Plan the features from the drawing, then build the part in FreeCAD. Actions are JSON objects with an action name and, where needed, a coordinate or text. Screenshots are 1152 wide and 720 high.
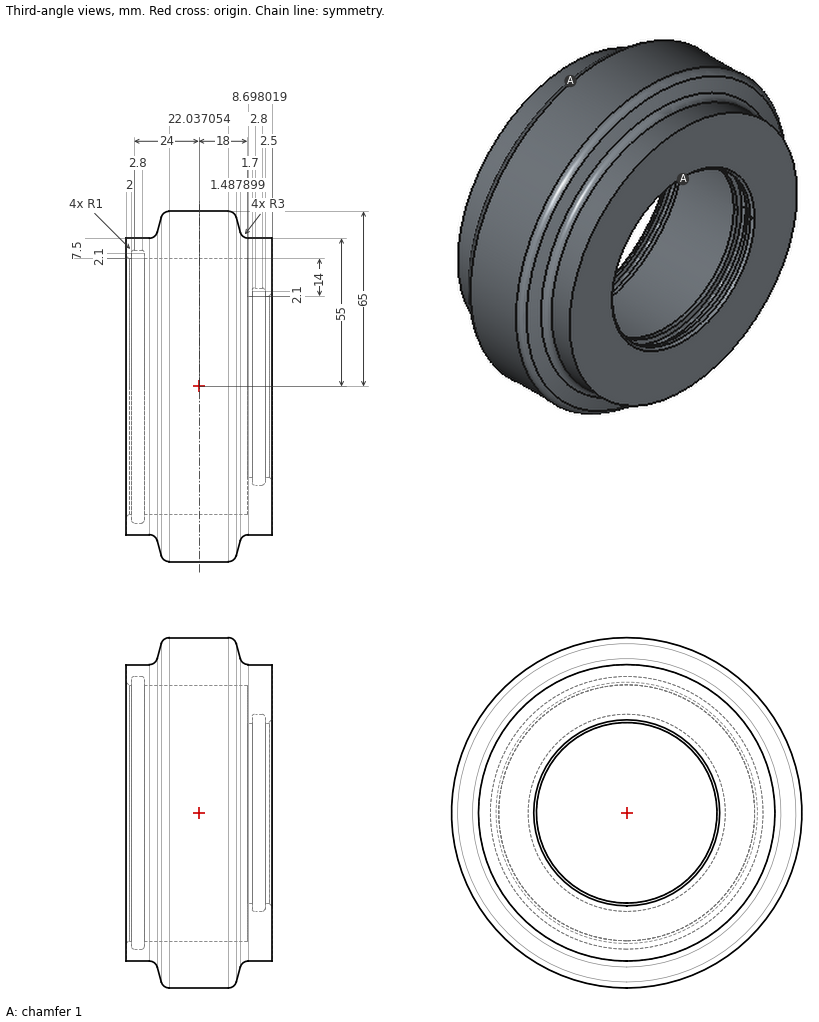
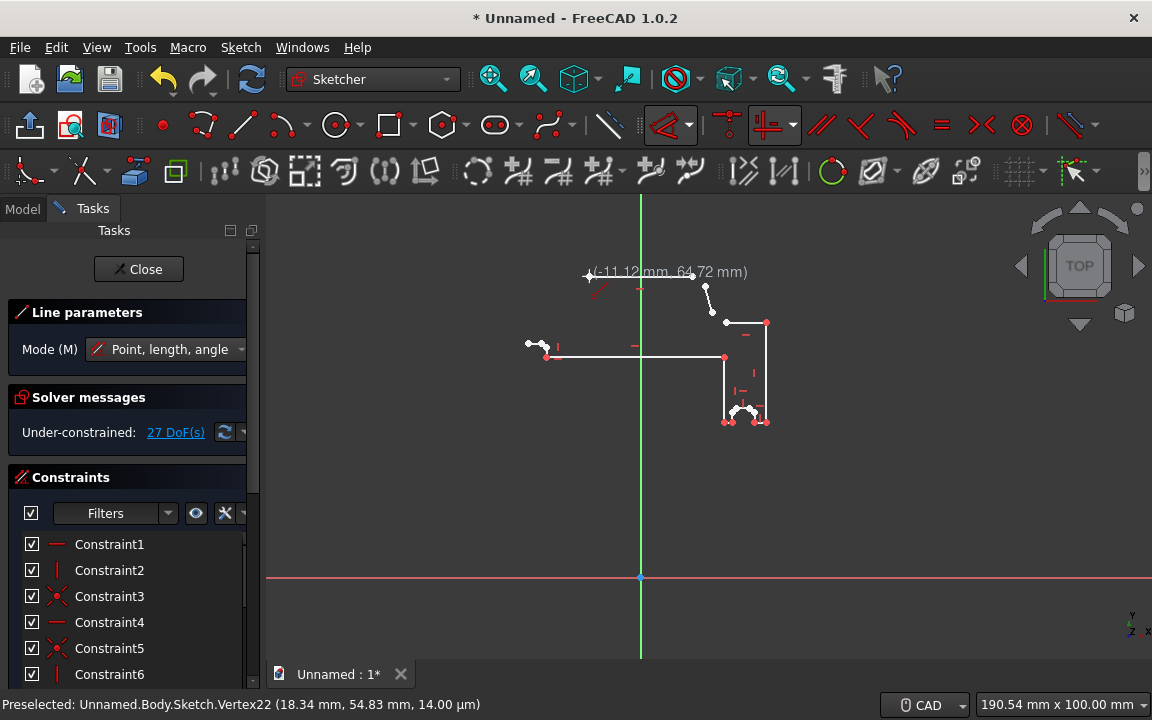
{"action": "left_click", "coordinate": [576, 286]}
{"action": "left_click", "coordinate": [569, 312]}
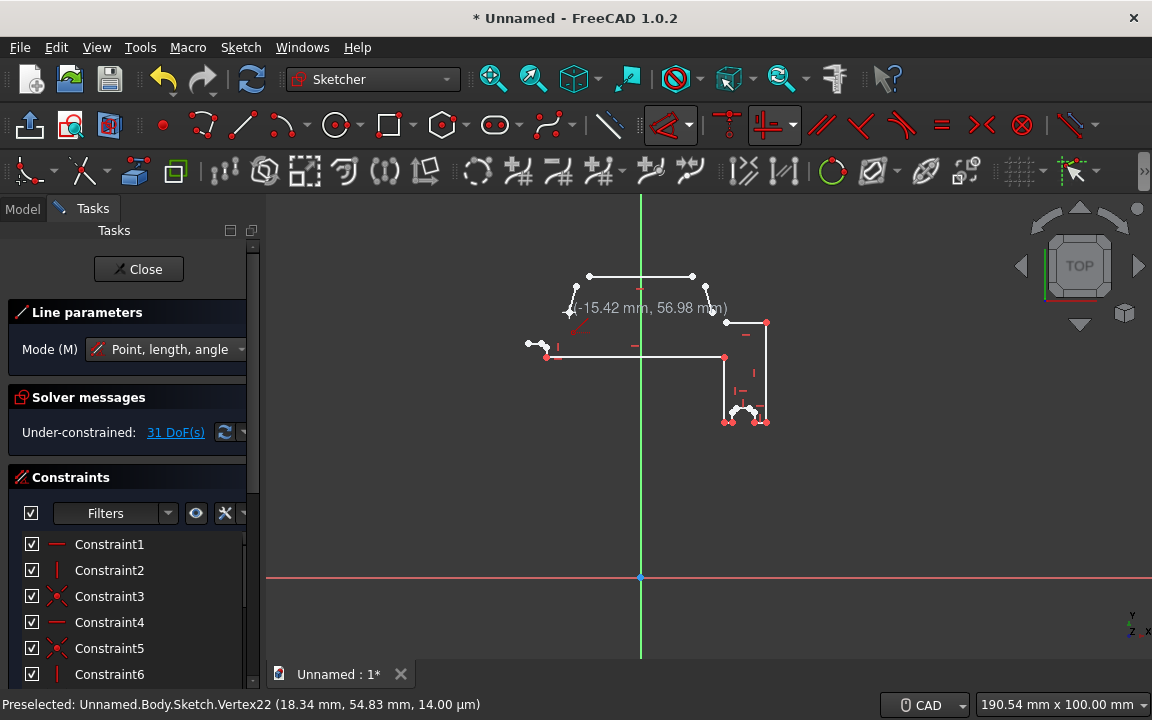
{"action": "key", "text": "g m"}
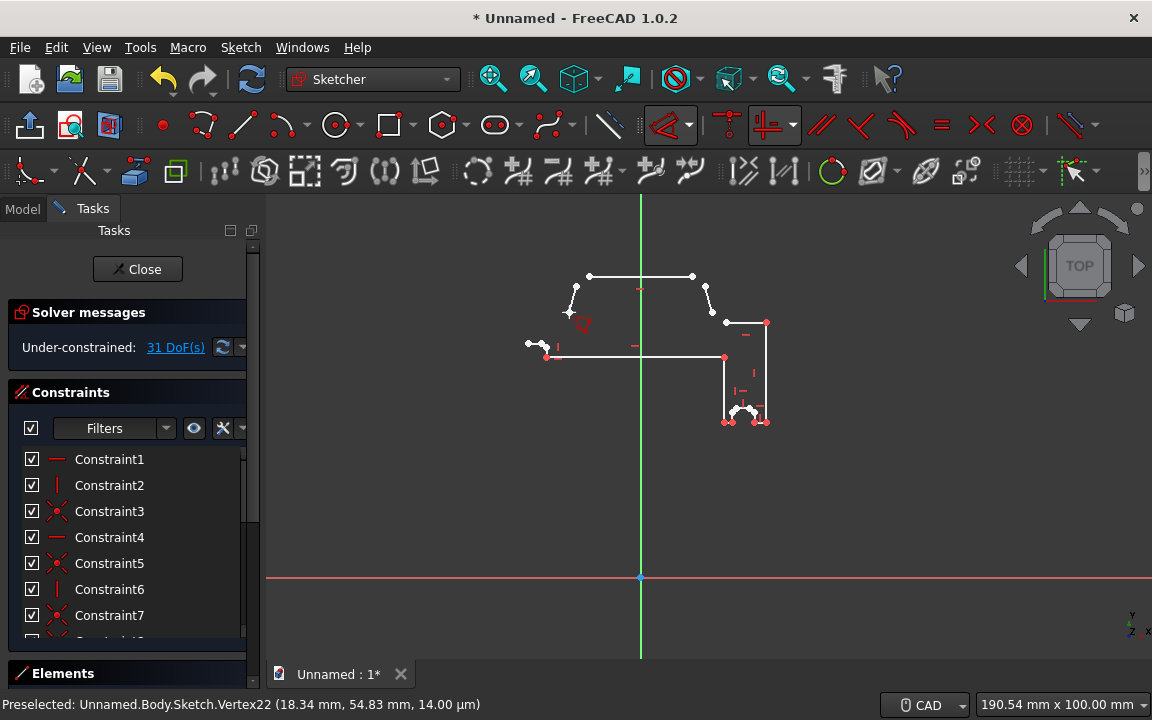
{"action": "left_click", "coordinate": [556, 322]}
{"action": "left_click", "coordinate": [515, 322]}
{"action": "left_click", "coordinate": [515, 357]}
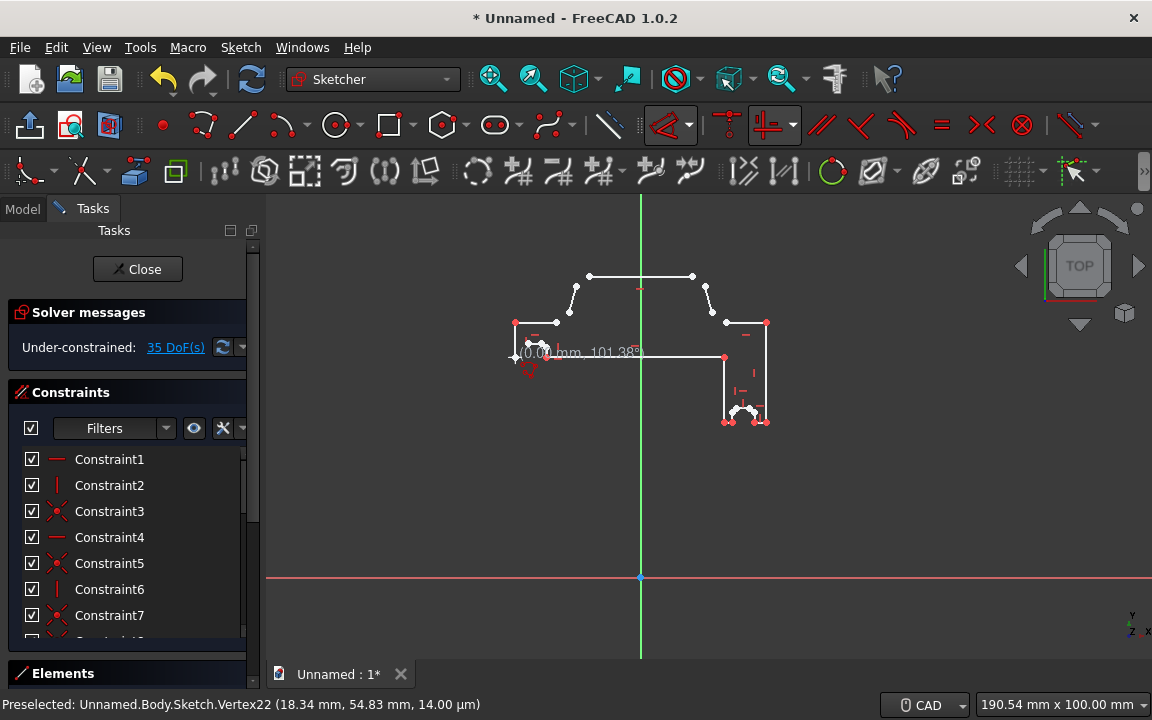
{"action": "scroll", "coordinate": [524, 357], "scroll_direction": "up", "scroll_amount": 3}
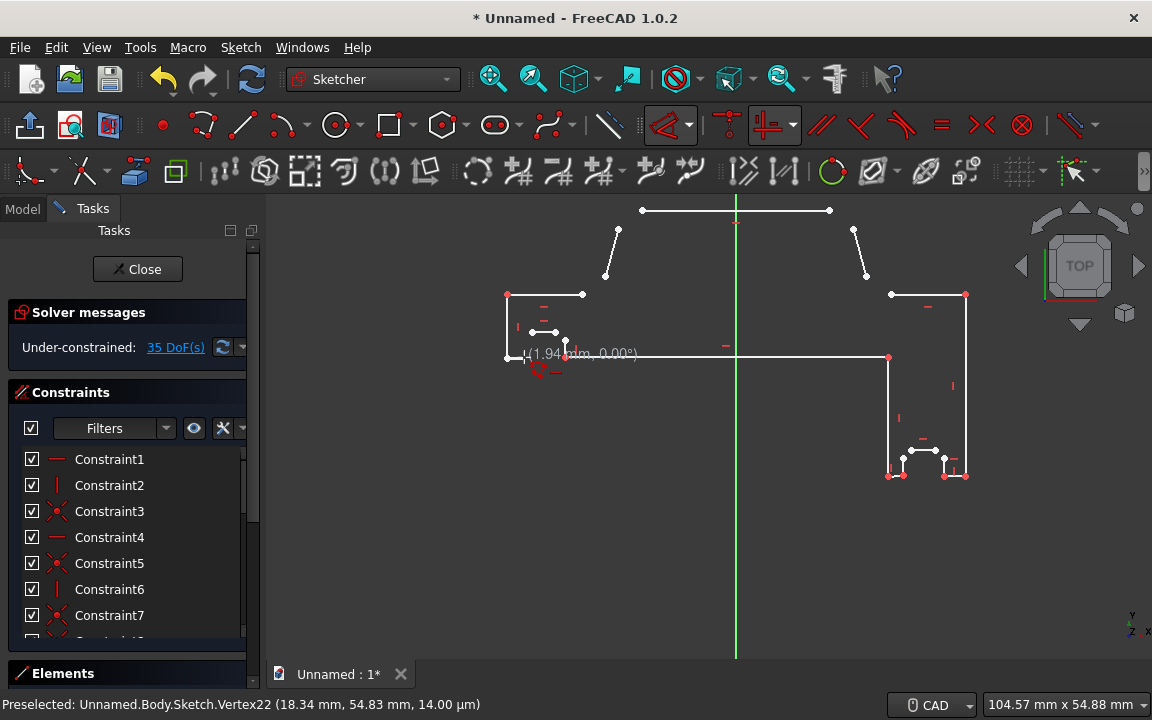
{"action": "left_click", "coordinate": [525, 357]}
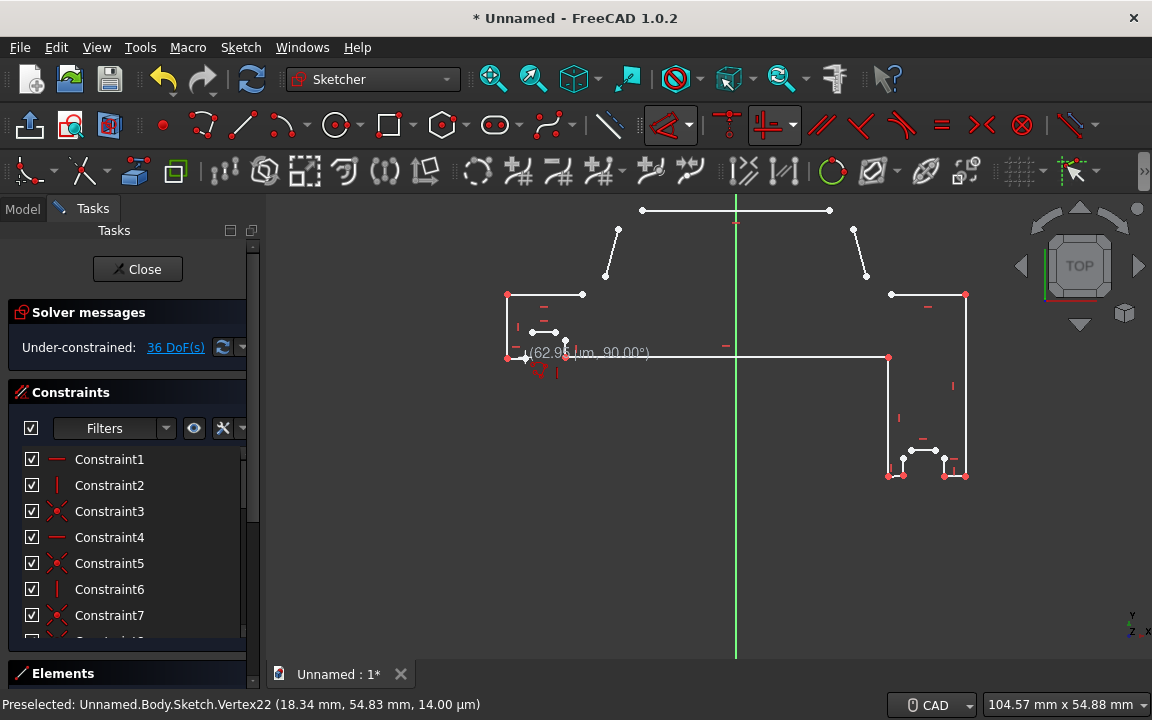
{"action": "scroll", "coordinate": [525, 339], "scroll_direction": "up", "scroll_amount": 2}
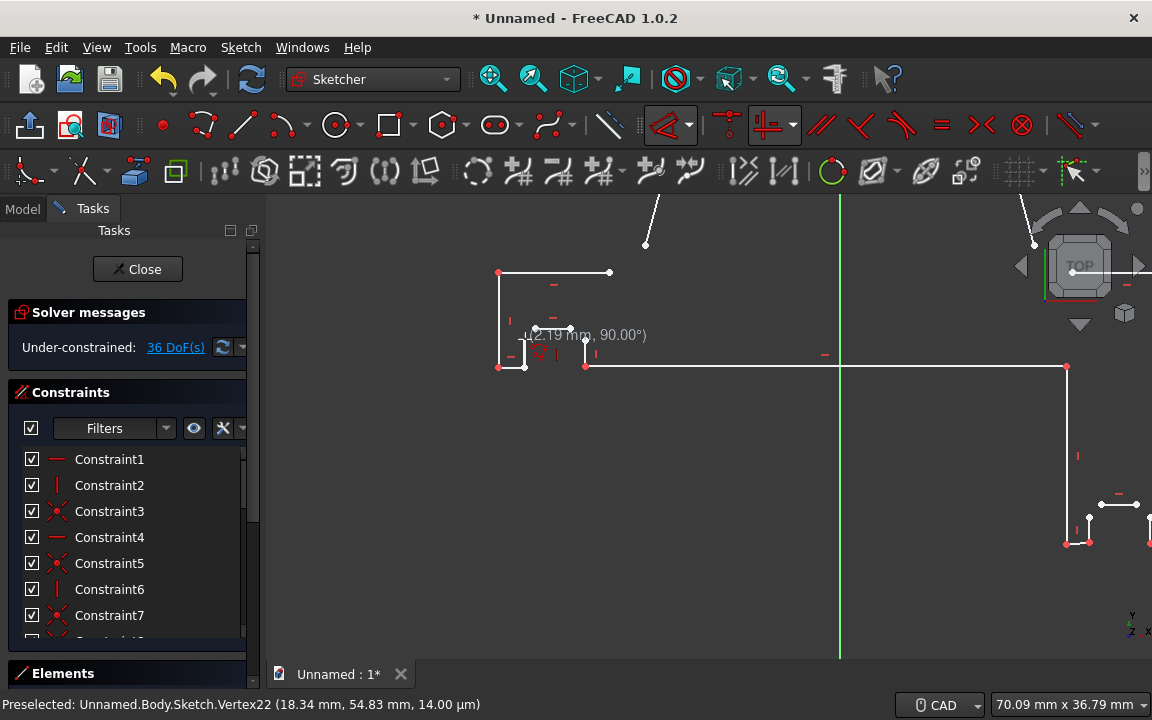
{"action": "left_click", "coordinate": [525, 339]}
{"action": "right_click", "coordinate": [525, 339]}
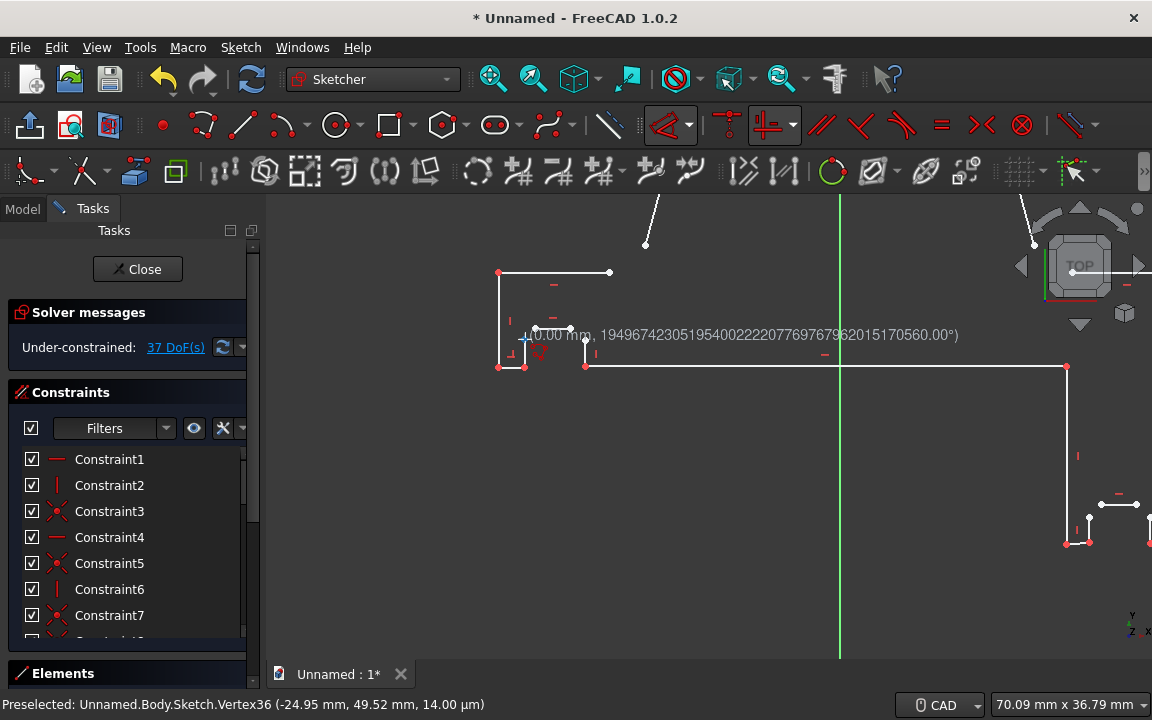
{"action": "key", "text": "g 3 a"}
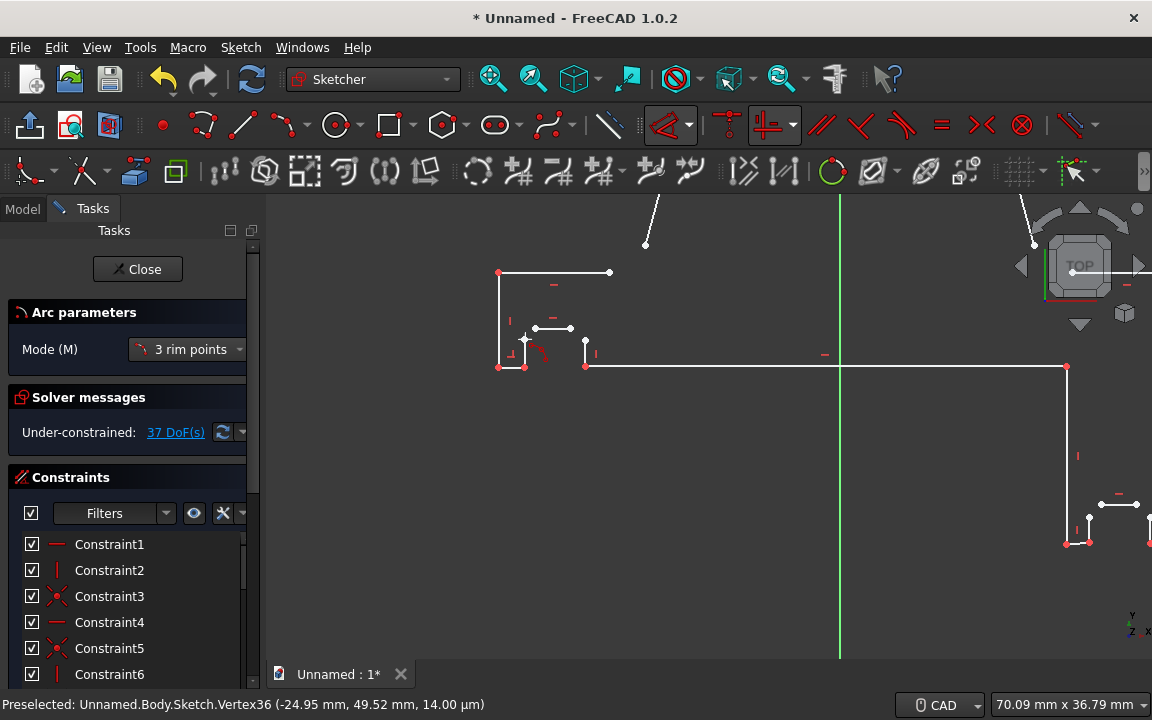
{"action": "left_click", "coordinate": [571, 329]}
{"action": "left_click", "coordinate": [585, 340]}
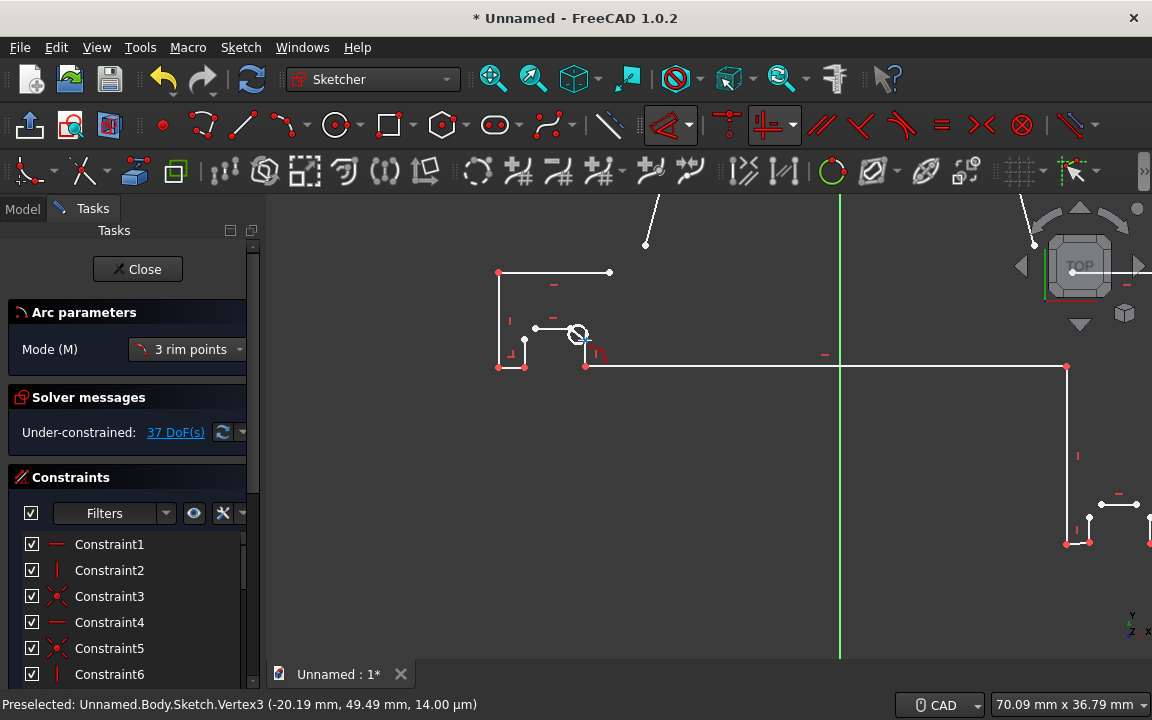
{"action": "scroll", "coordinate": [581, 330], "scroll_direction": "up", "scroll_amount": 8}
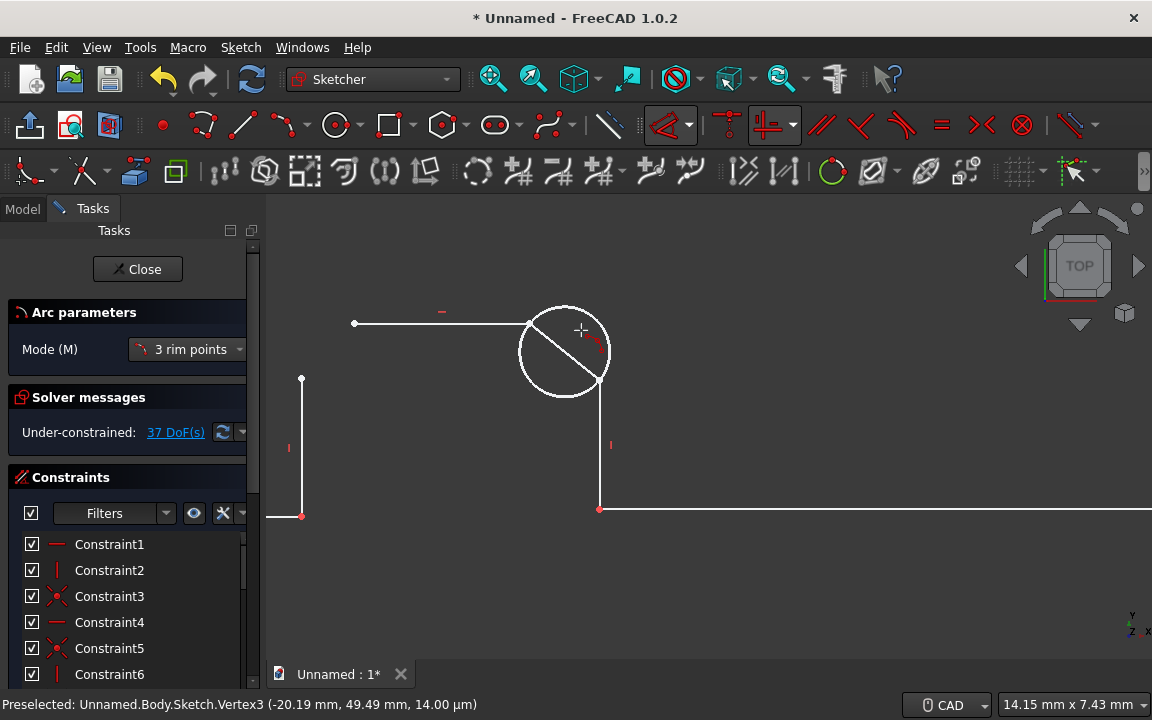
{"action": "left_click", "coordinate": [581, 329]}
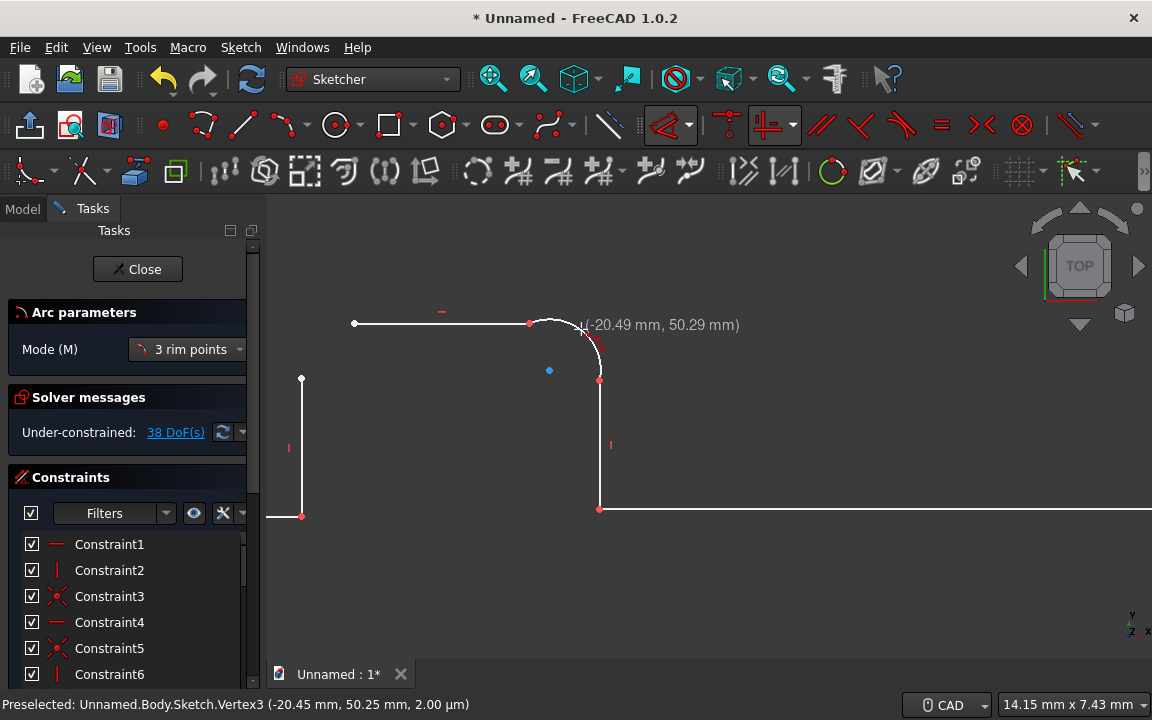
{"action": "scroll", "coordinate": [542, 345], "scroll_direction": "down", "scroll_amount": 13}